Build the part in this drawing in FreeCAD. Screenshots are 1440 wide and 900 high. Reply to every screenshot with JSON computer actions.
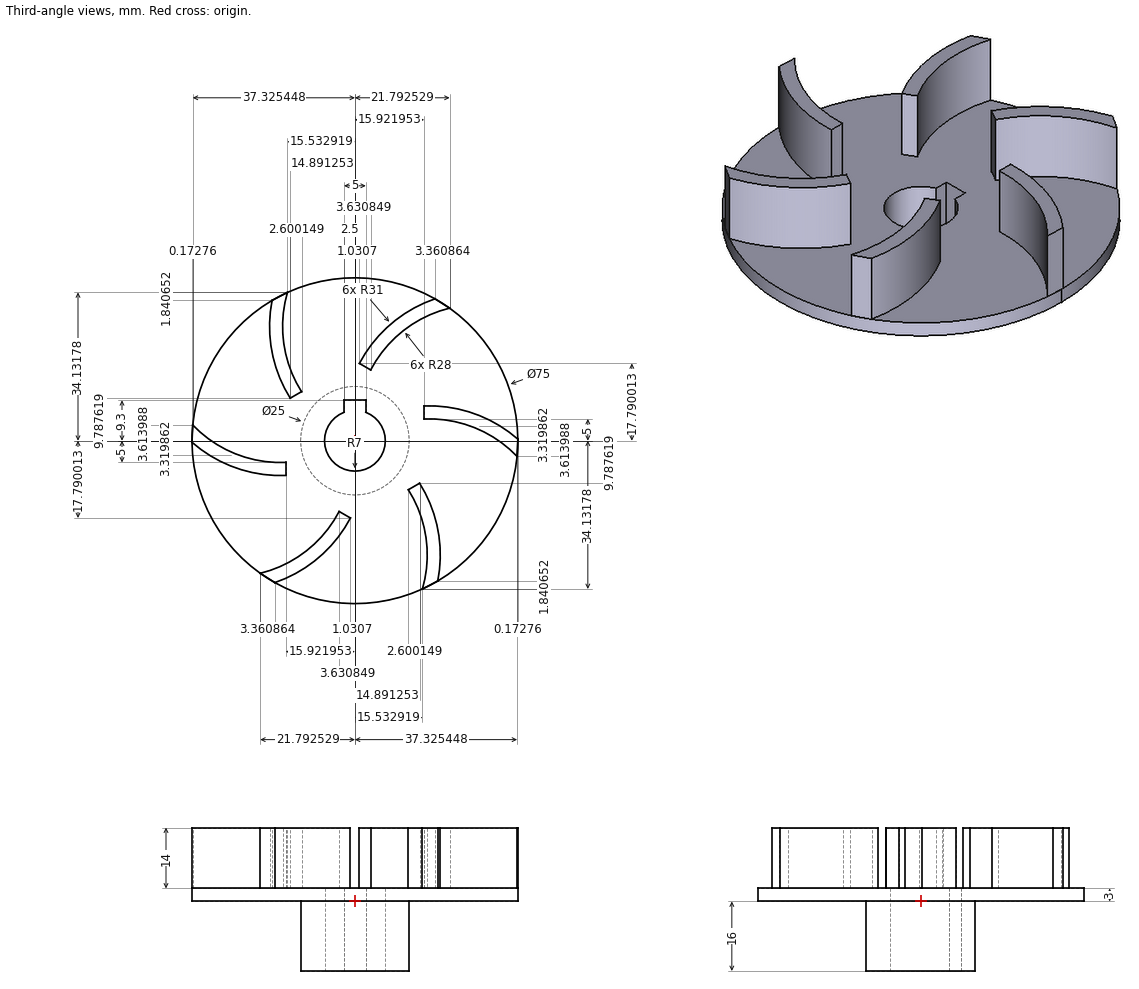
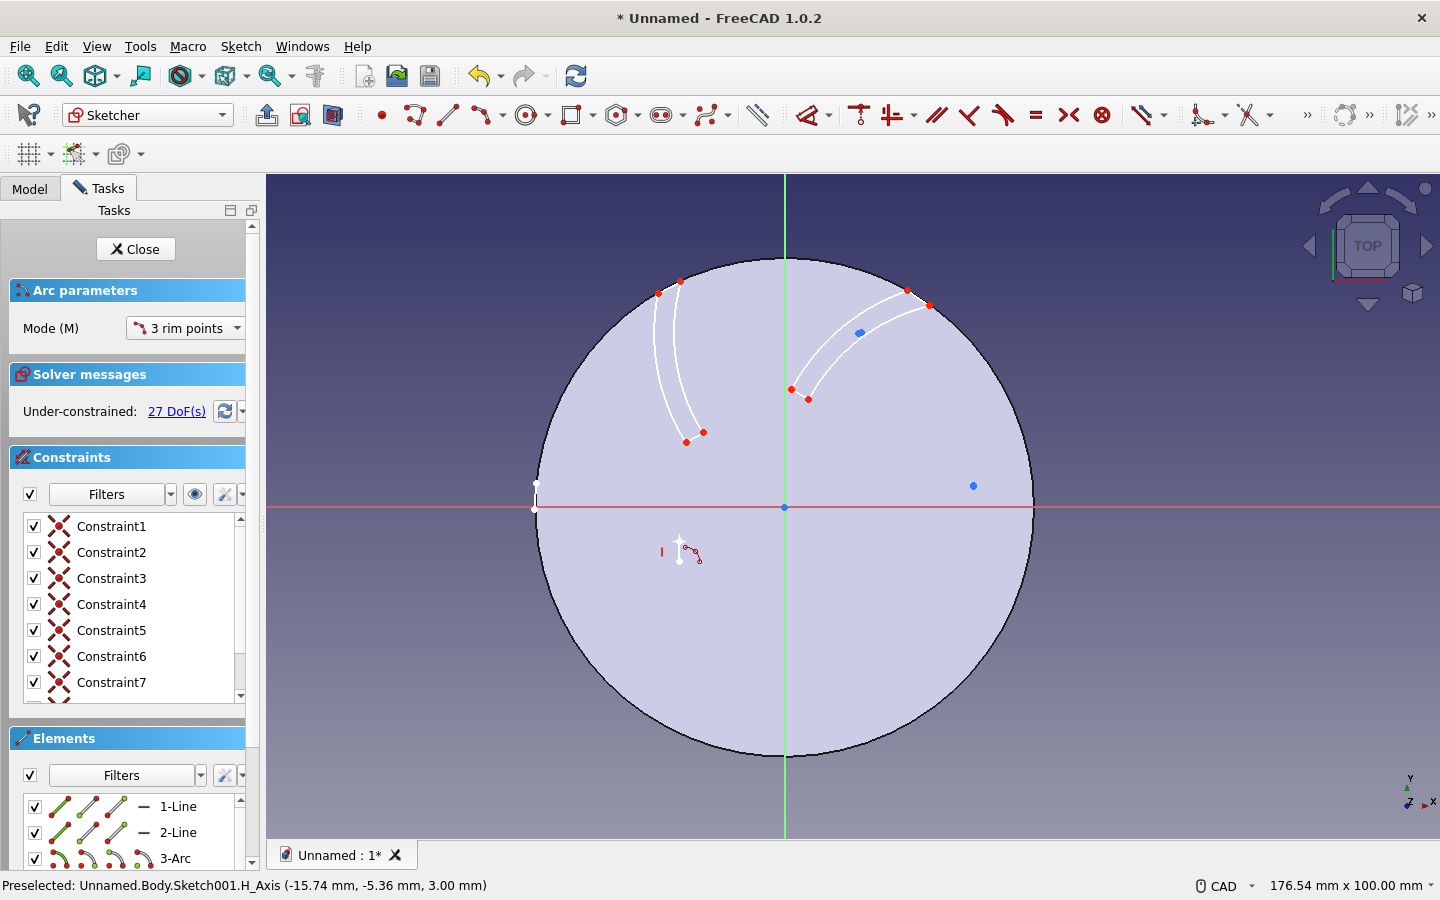
{"action": "scroll", "coordinate": [535, 510], "scroll_direction": "up", "scroll_amount": 10}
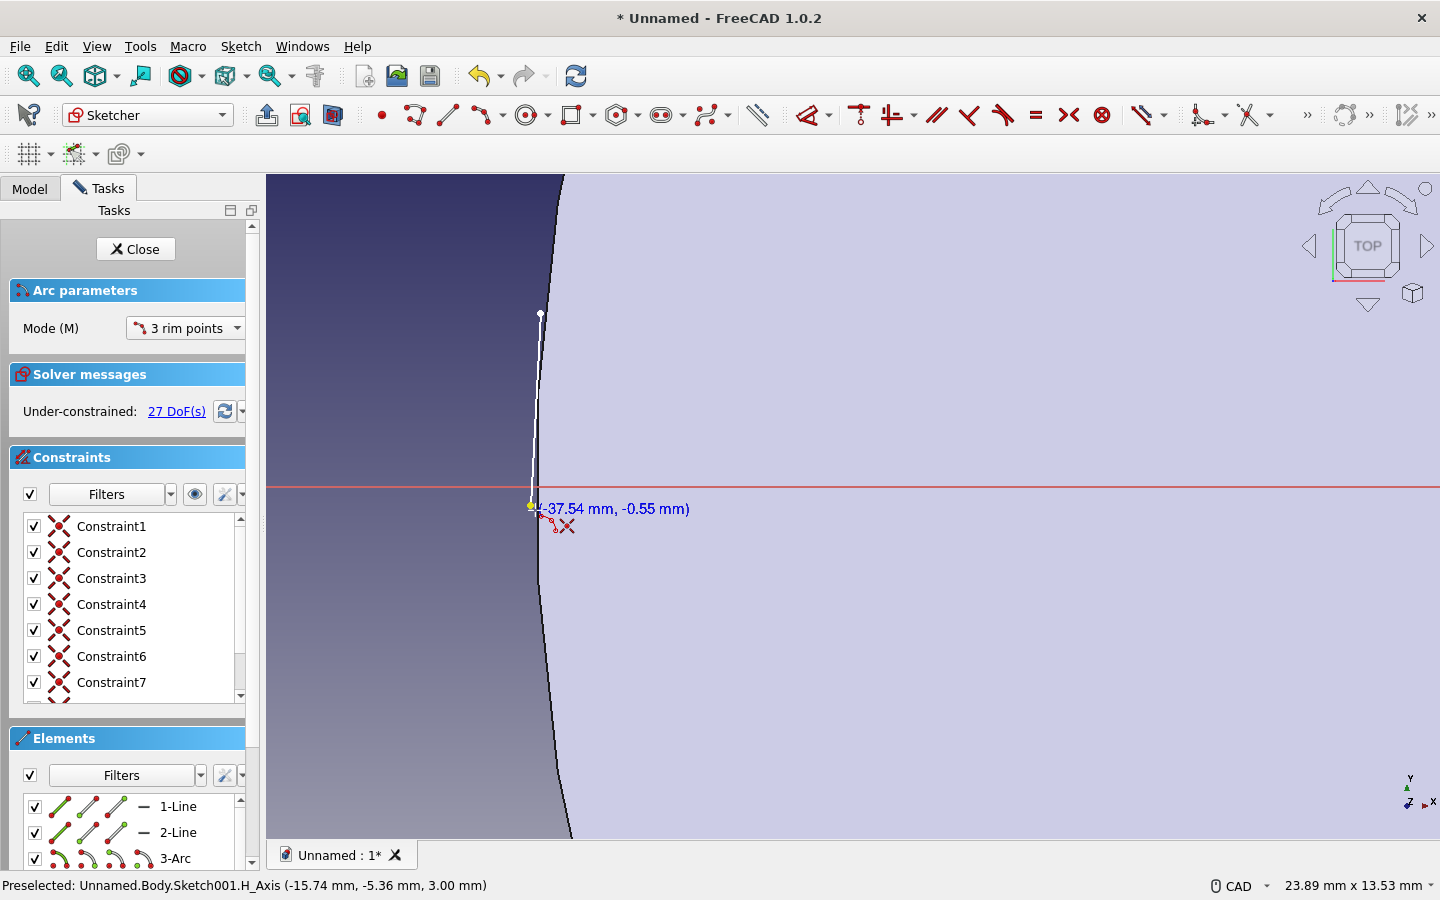
{"action": "left_click", "coordinate": [531, 506]}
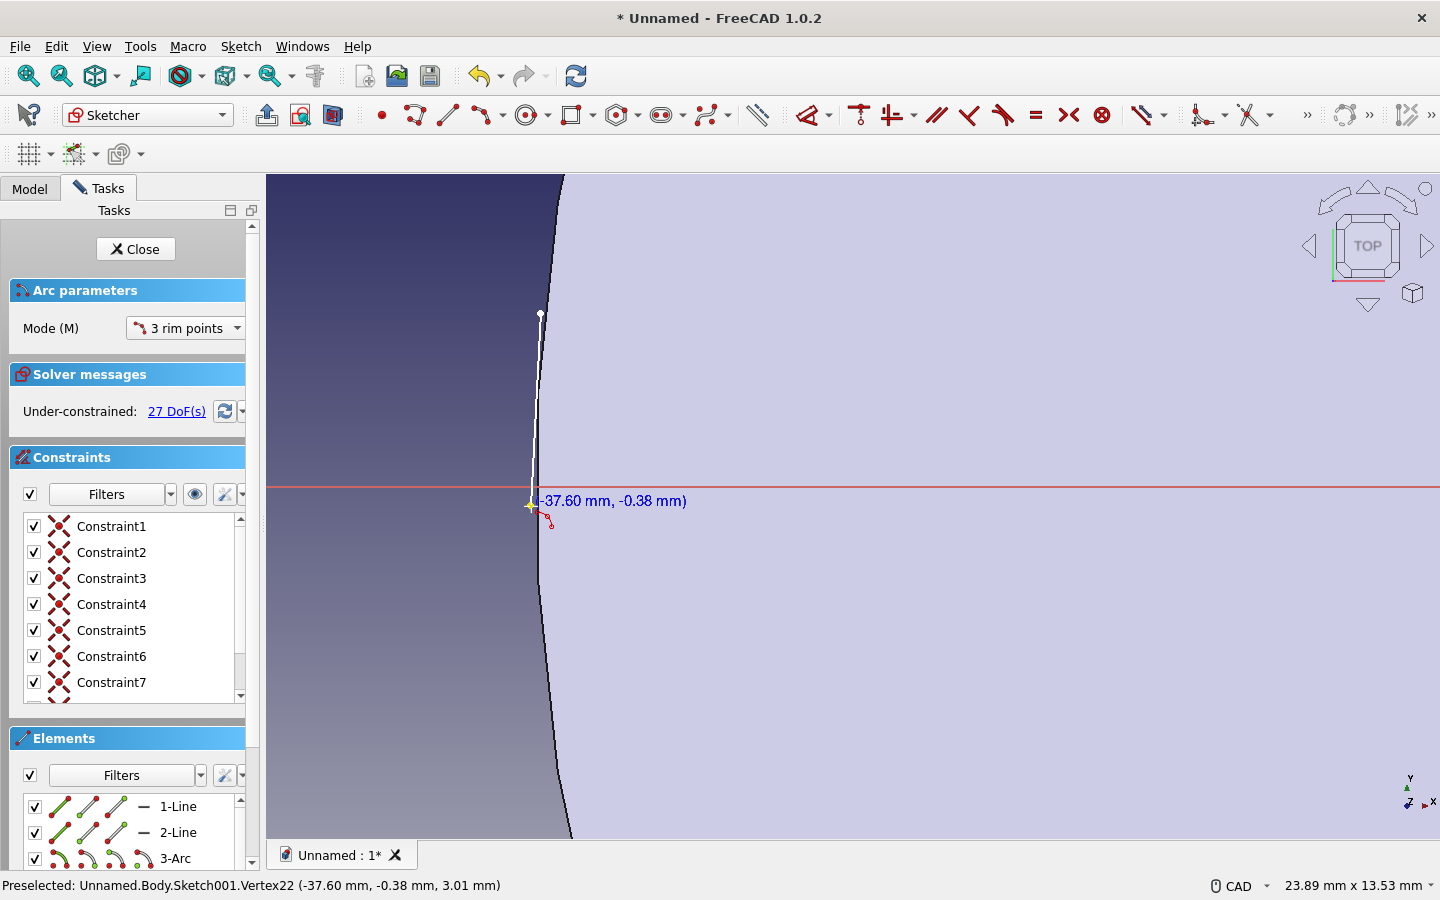
{"action": "scroll", "coordinate": [535, 510], "scroll_direction": "down", "scroll_amount": 10}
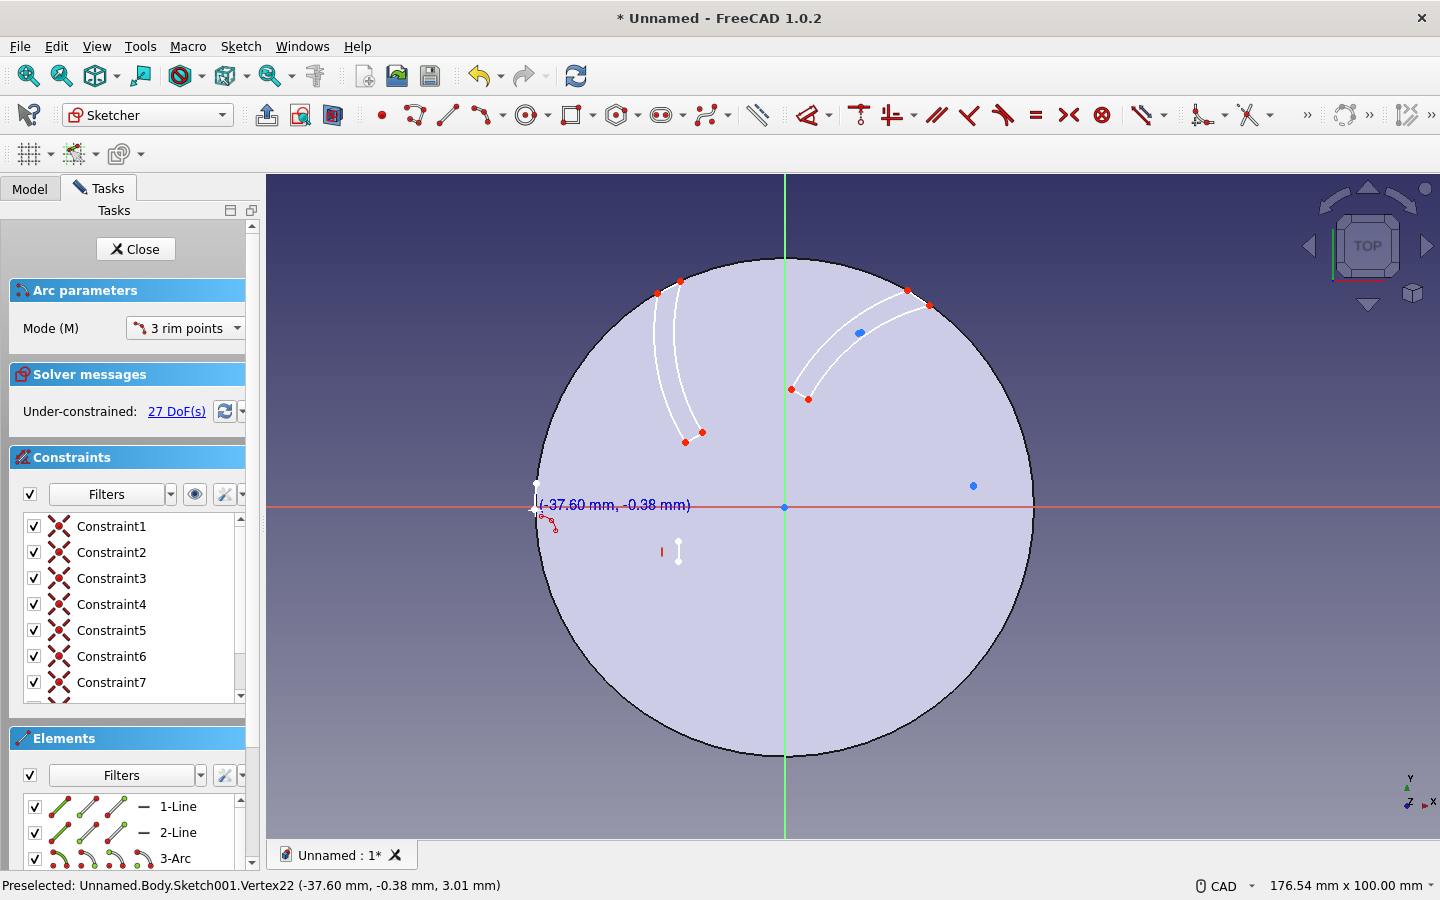
{"action": "scroll", "coordinate": [679, 561], "scroll_direction": "up", "scroll_amount": 3}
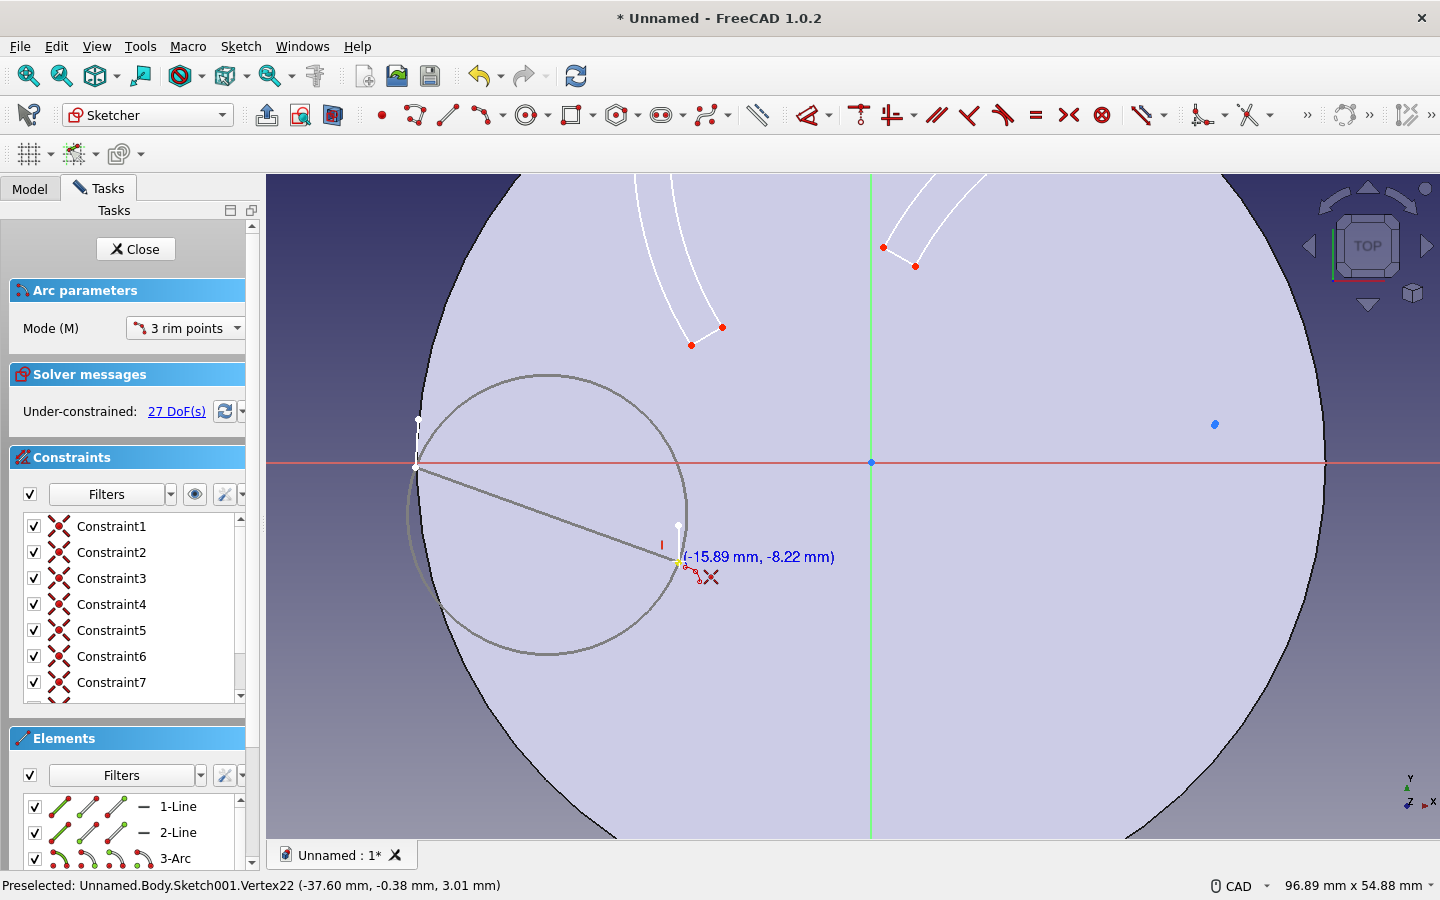
{"action": "left_click", "coordinate": [679, 562]}
{"action": "left_click", "coordinate": [539, 539]}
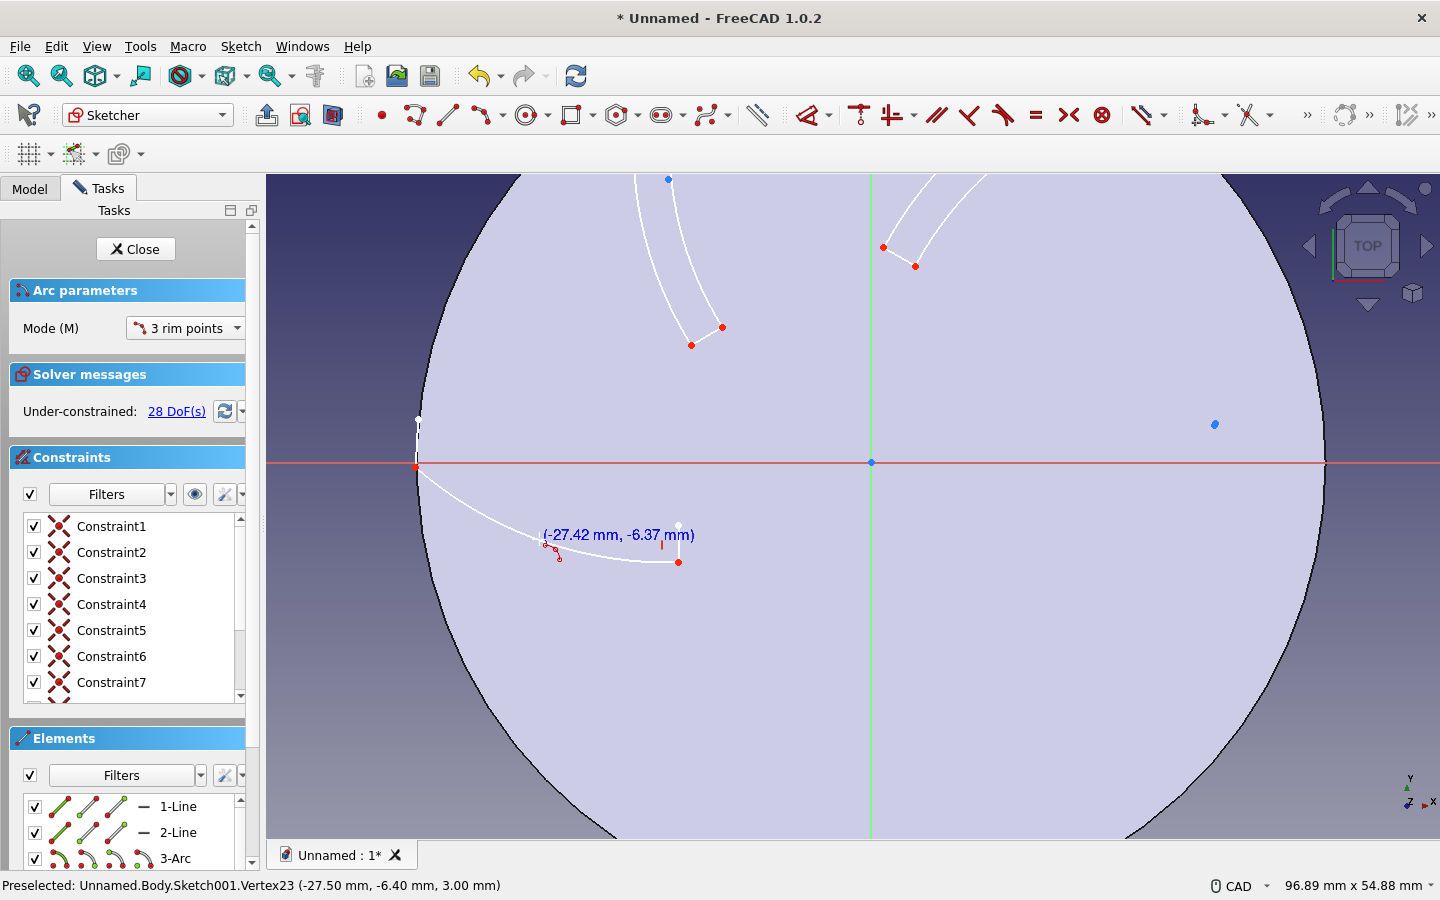
{"action": "left_click", "coordinate": [679, 526]}
{"action": "left_click", "coordinate": [418, 420]}
{"action": "left_click", "coordinate": [537, 499]}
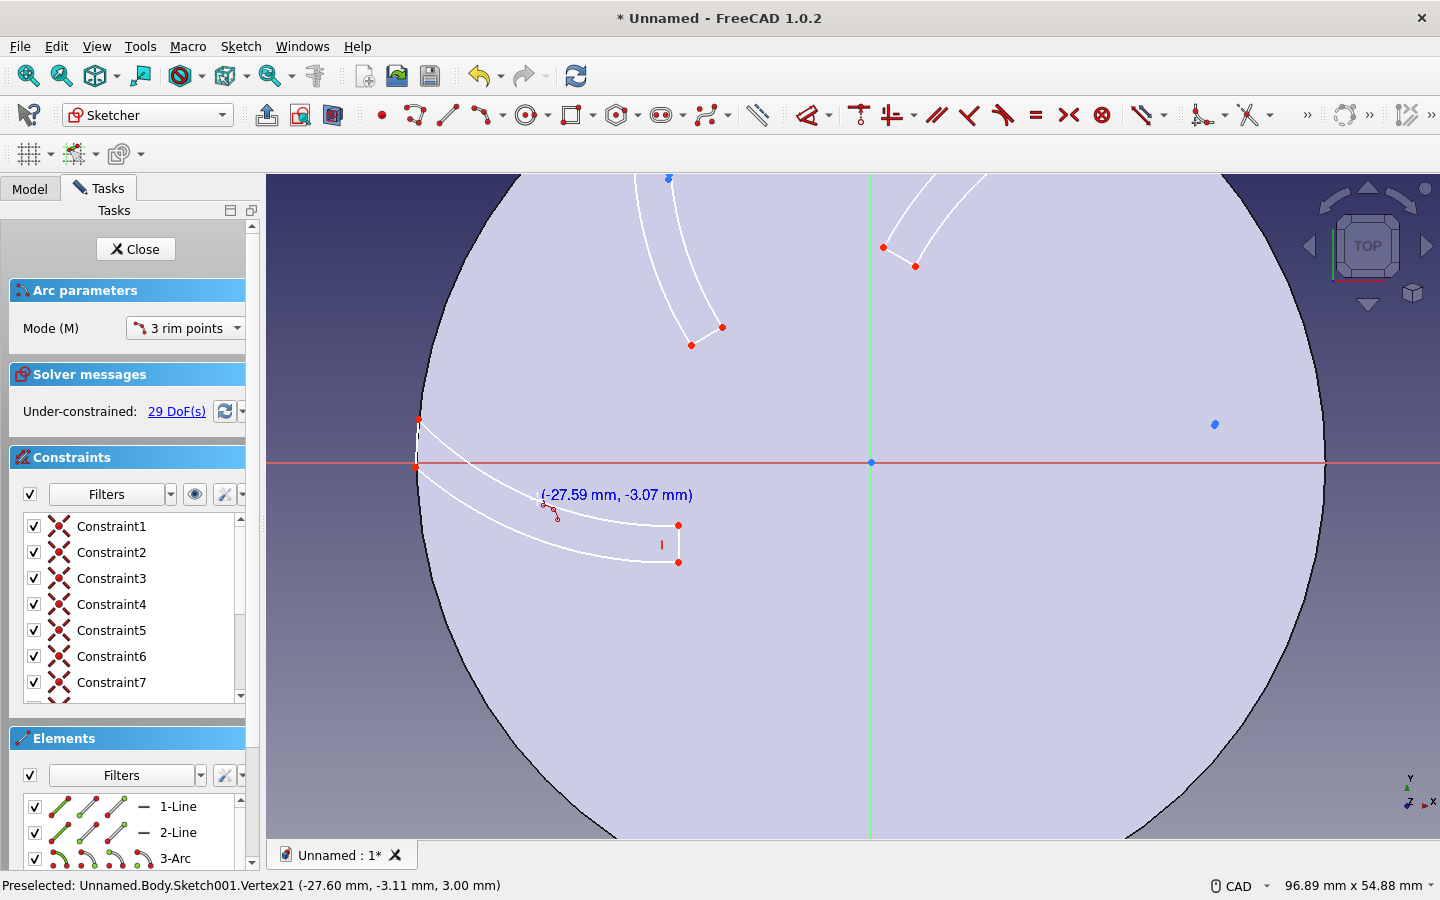
{"action": "key", "text": "g l"}